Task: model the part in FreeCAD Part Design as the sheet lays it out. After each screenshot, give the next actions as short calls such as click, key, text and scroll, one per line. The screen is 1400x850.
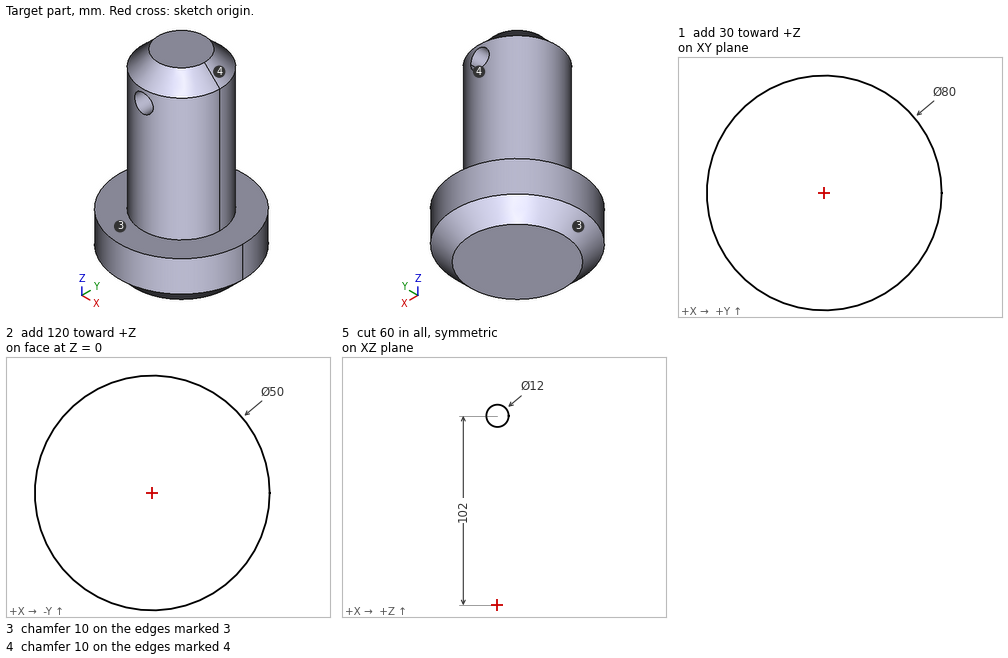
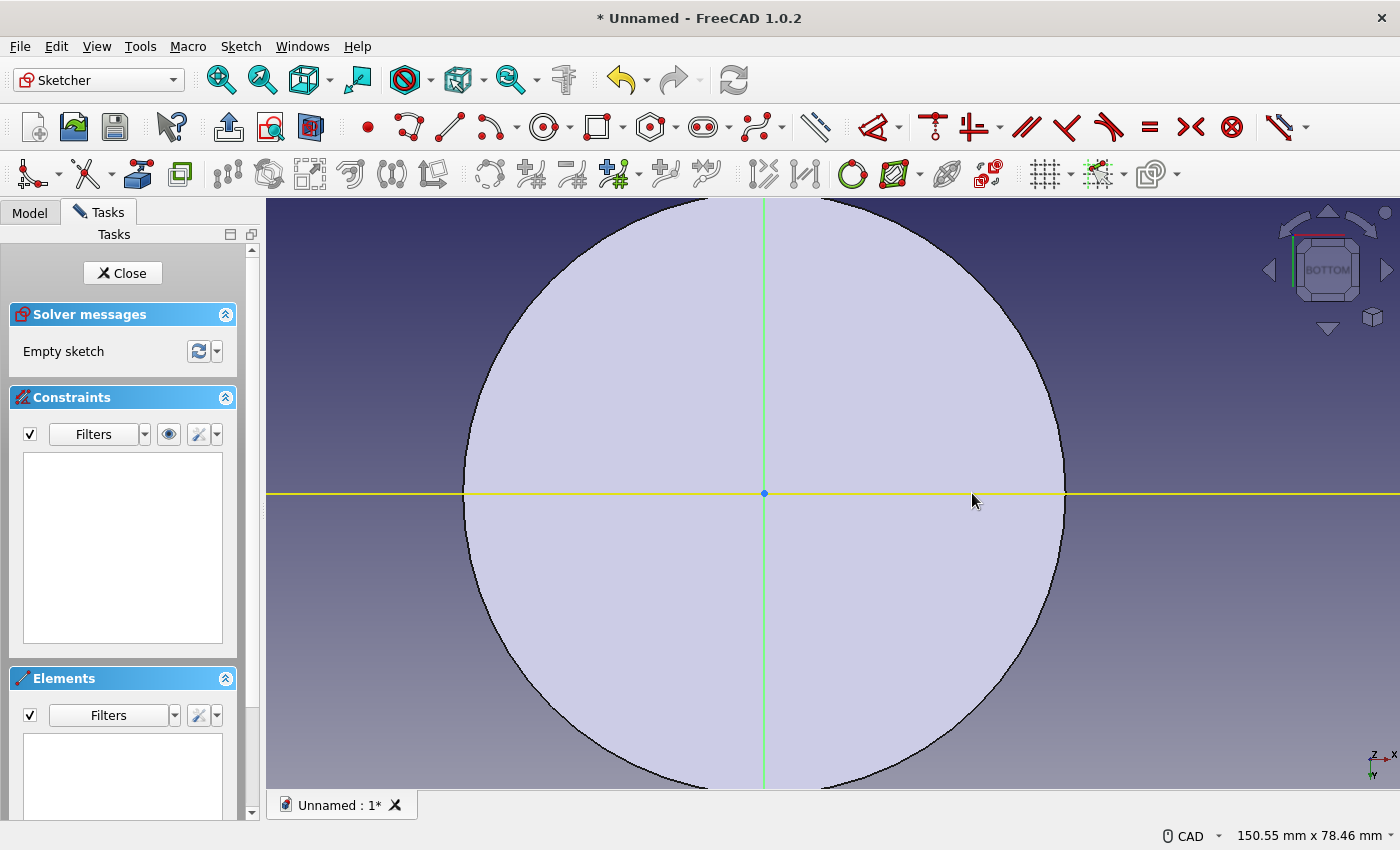
key(g)
key(c)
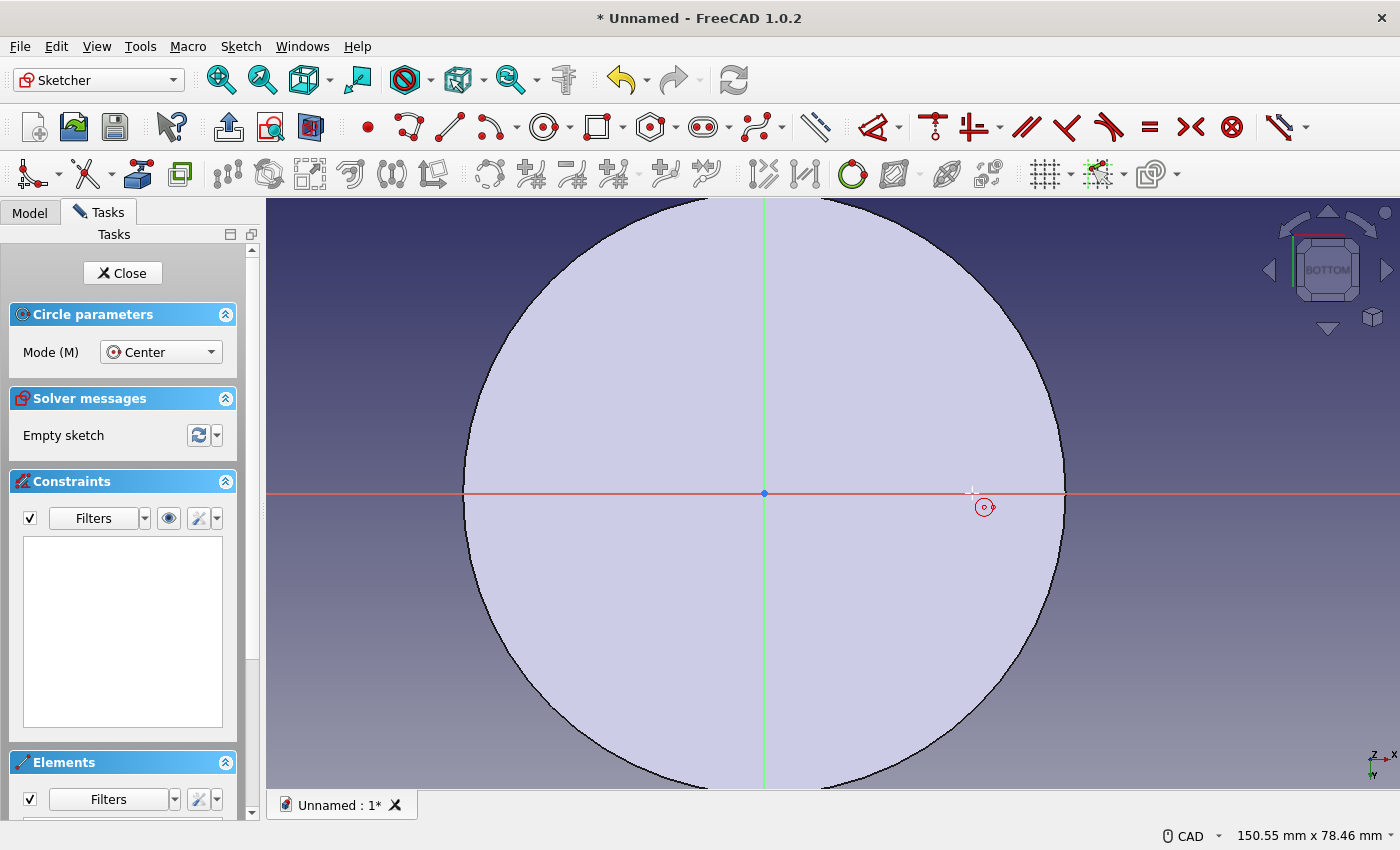
click(764, 494)
click(897, 360)
key(Escape)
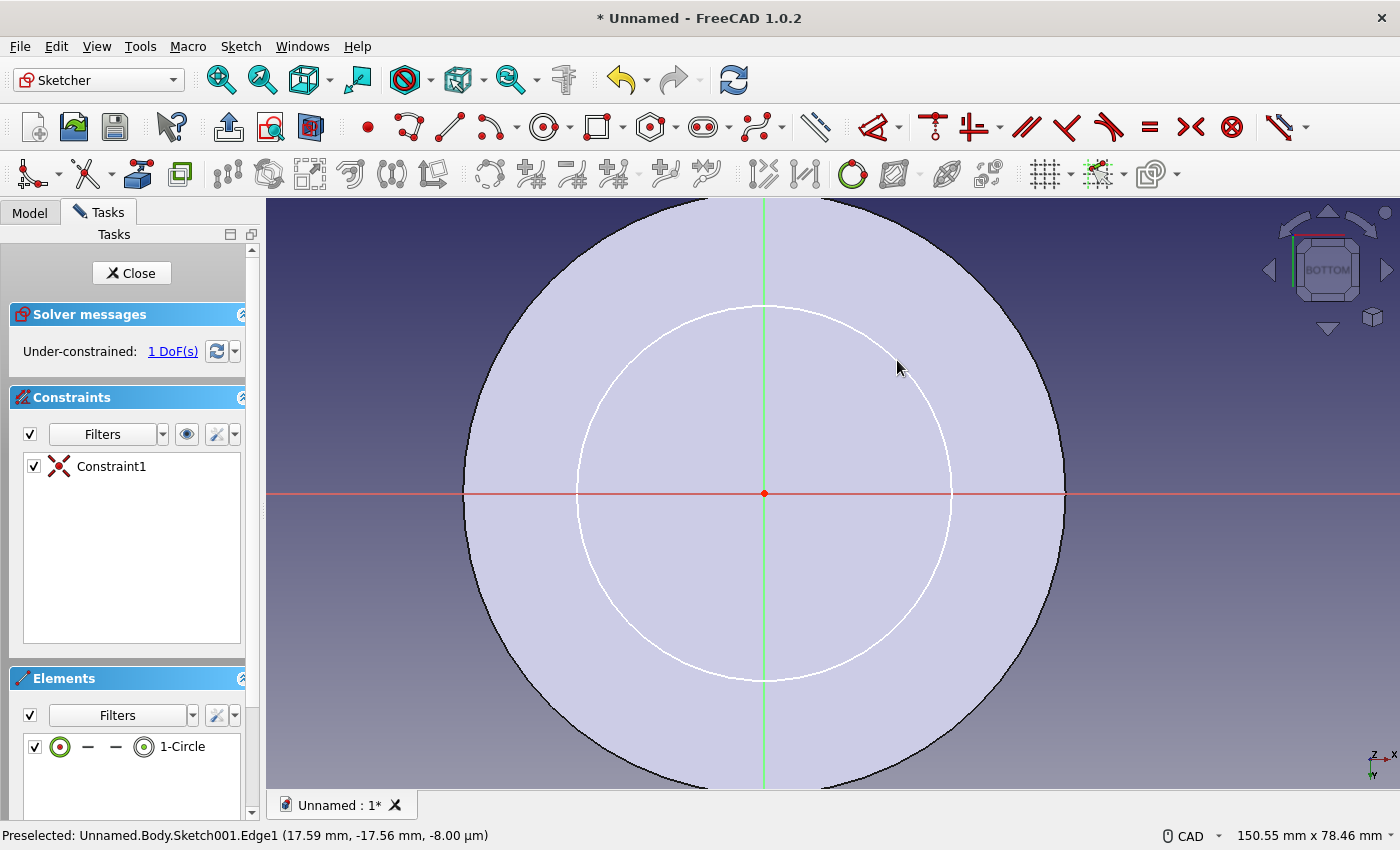
key(d)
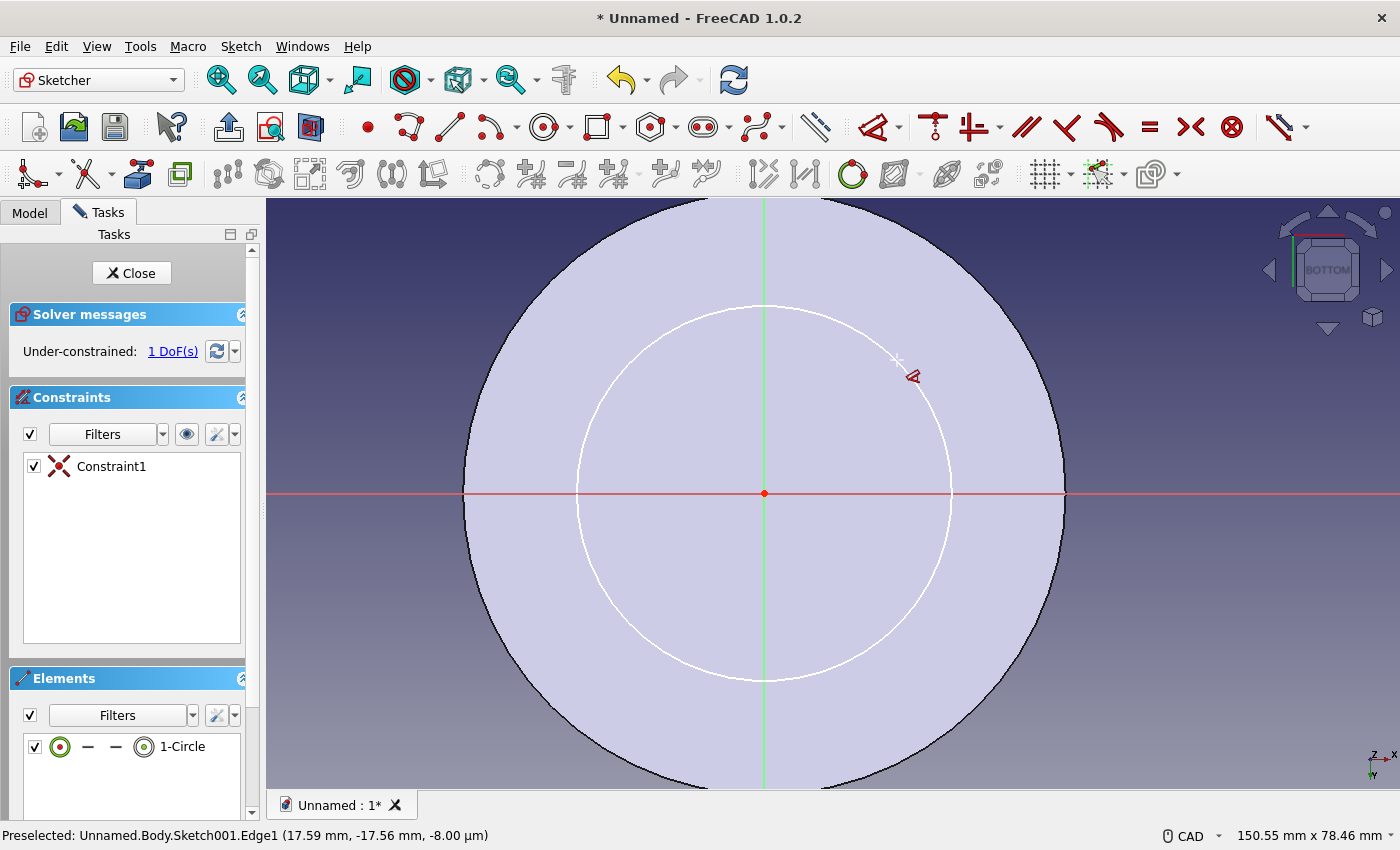
click(897, 361)
click(920, 338)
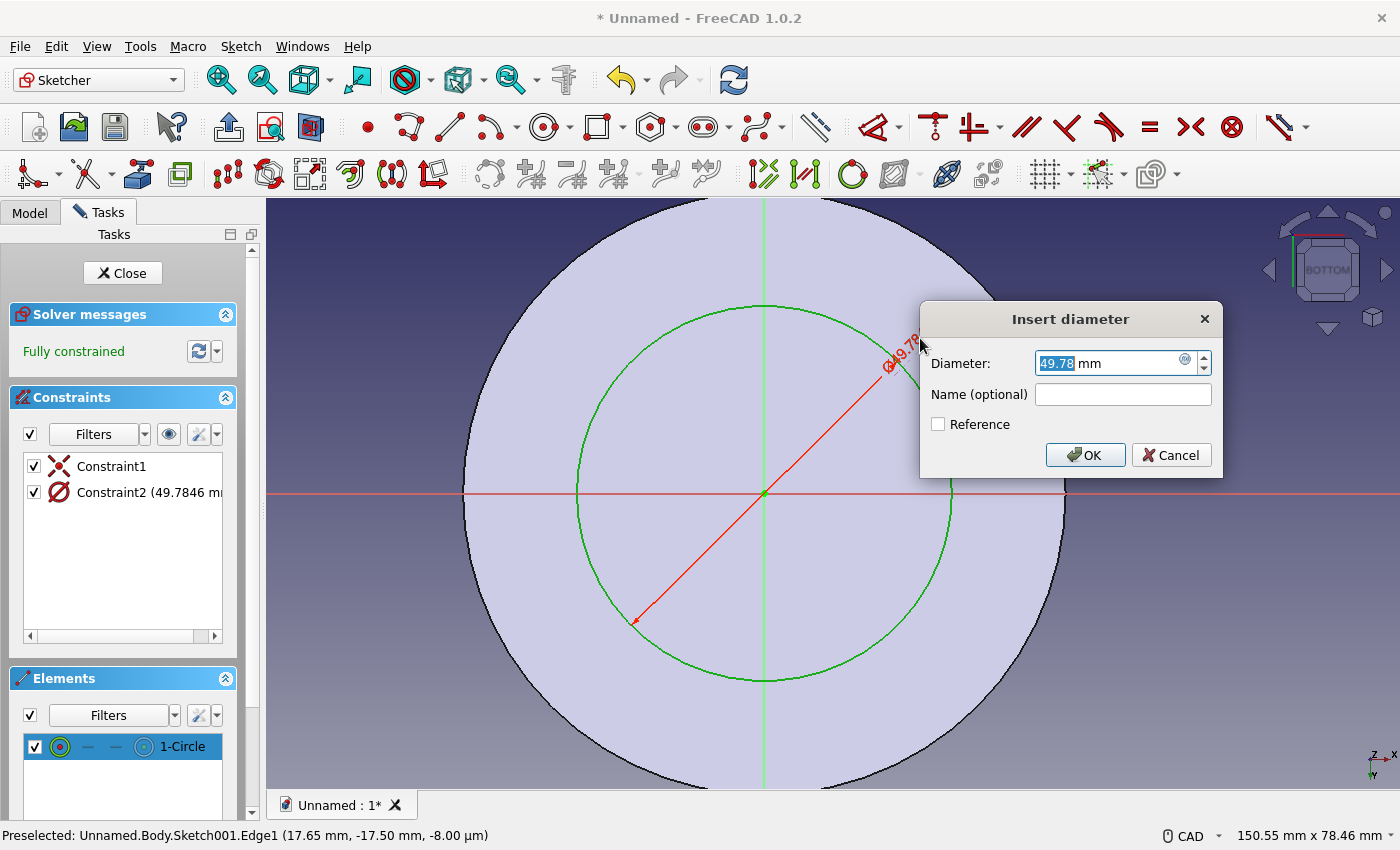
text(50)
key(Return)
key(Escape)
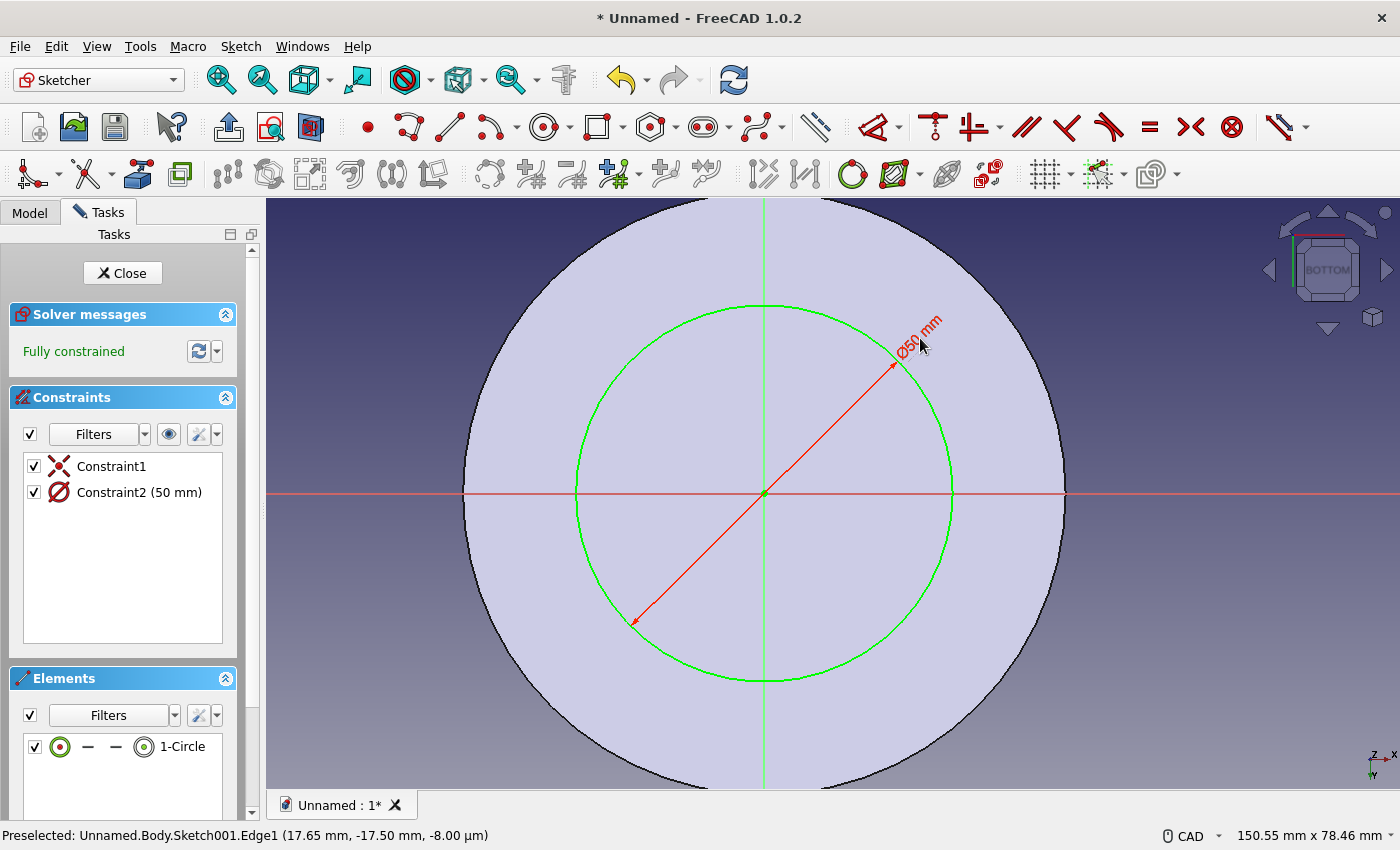
click(123, 273)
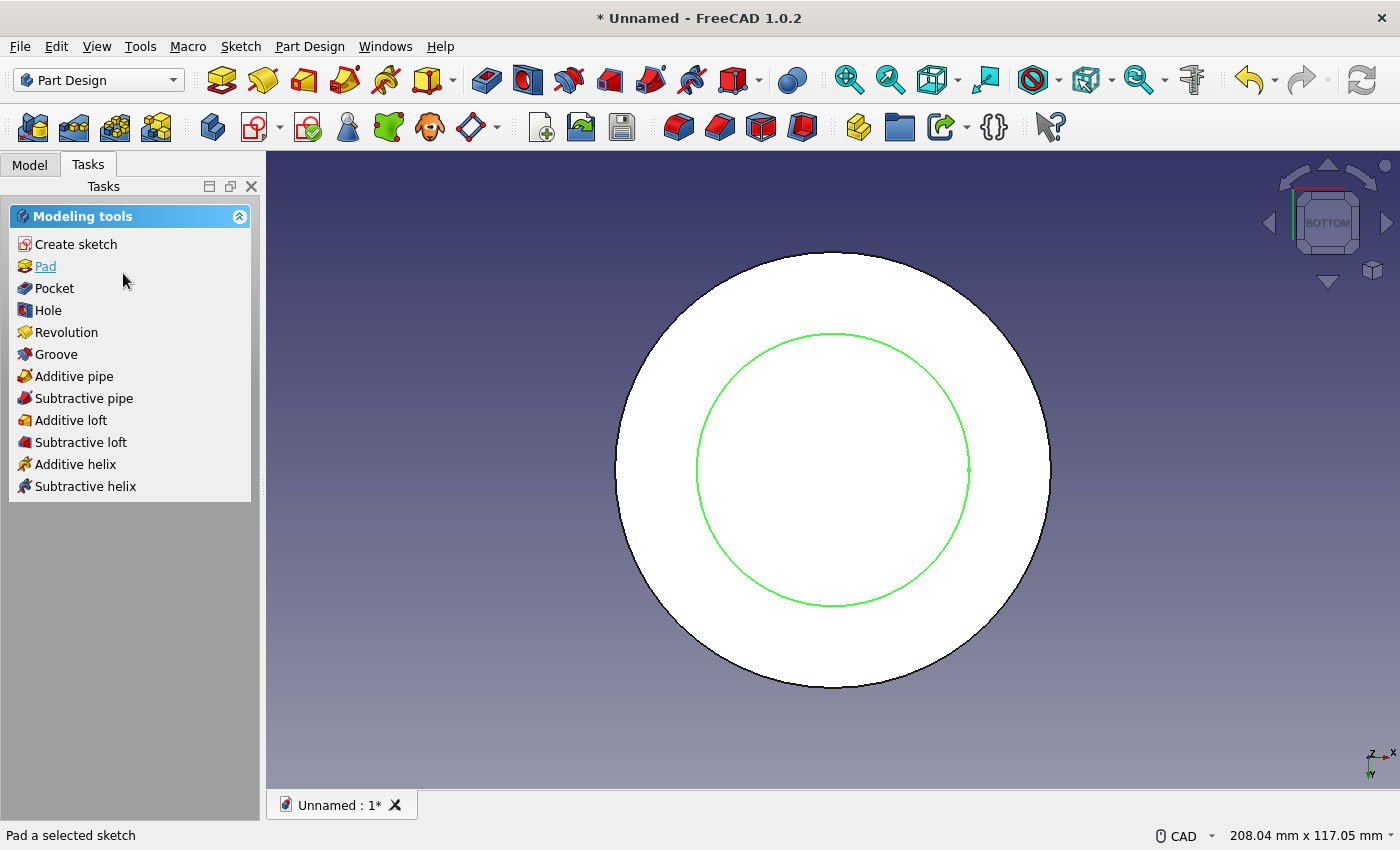
click(222, 80)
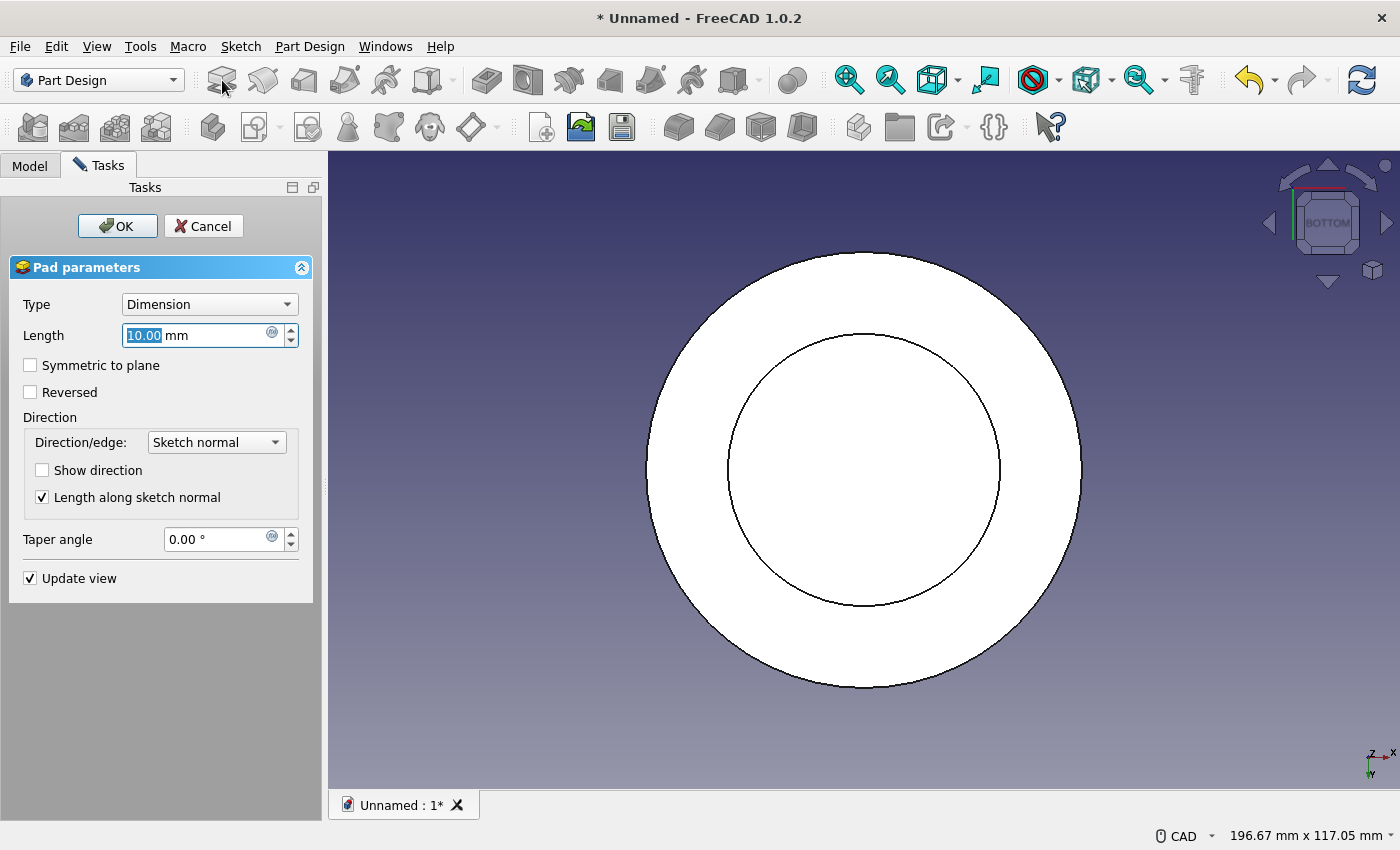
text(120)
key(Tab)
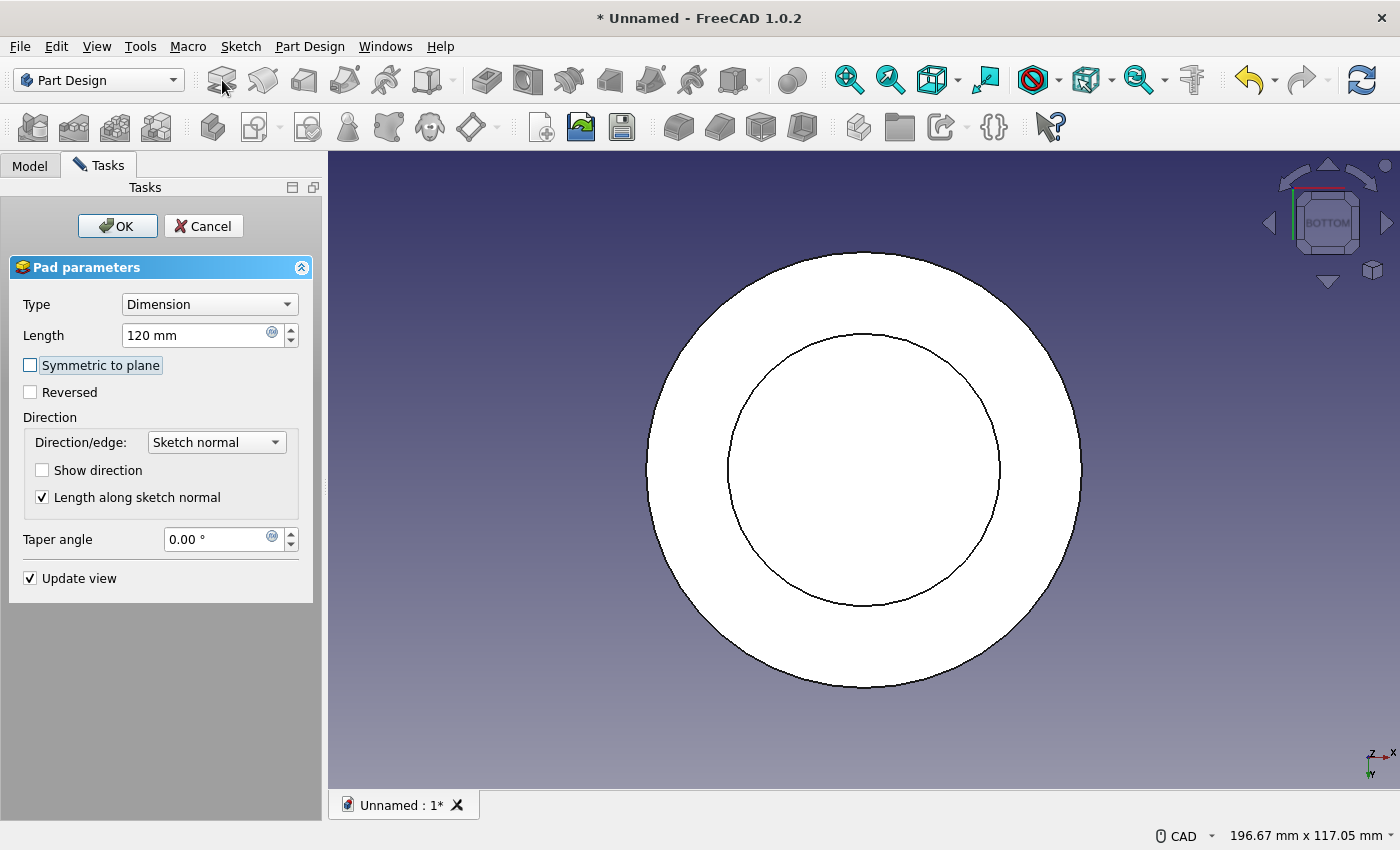
click(31, 392)